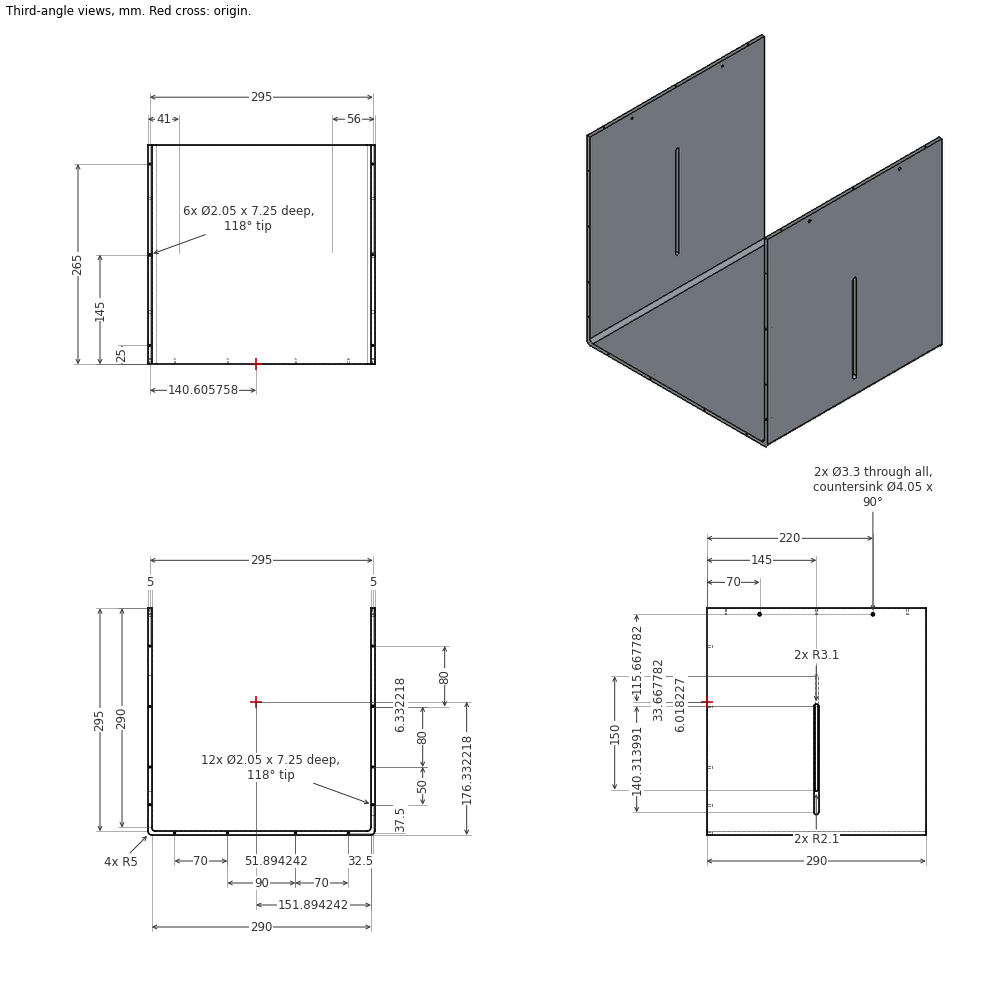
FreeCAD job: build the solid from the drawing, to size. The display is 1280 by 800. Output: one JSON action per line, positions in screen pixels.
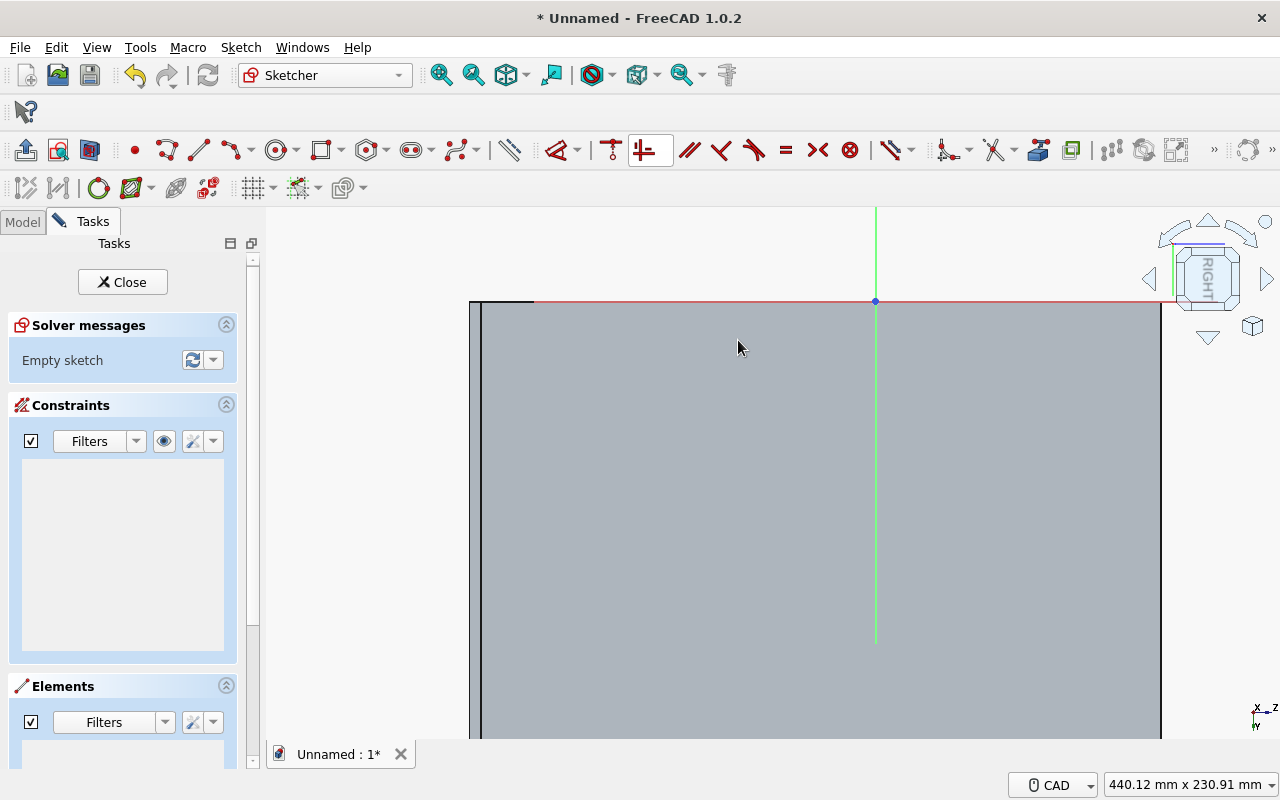
{"action": "left_click", "coordinate": [412, 150]}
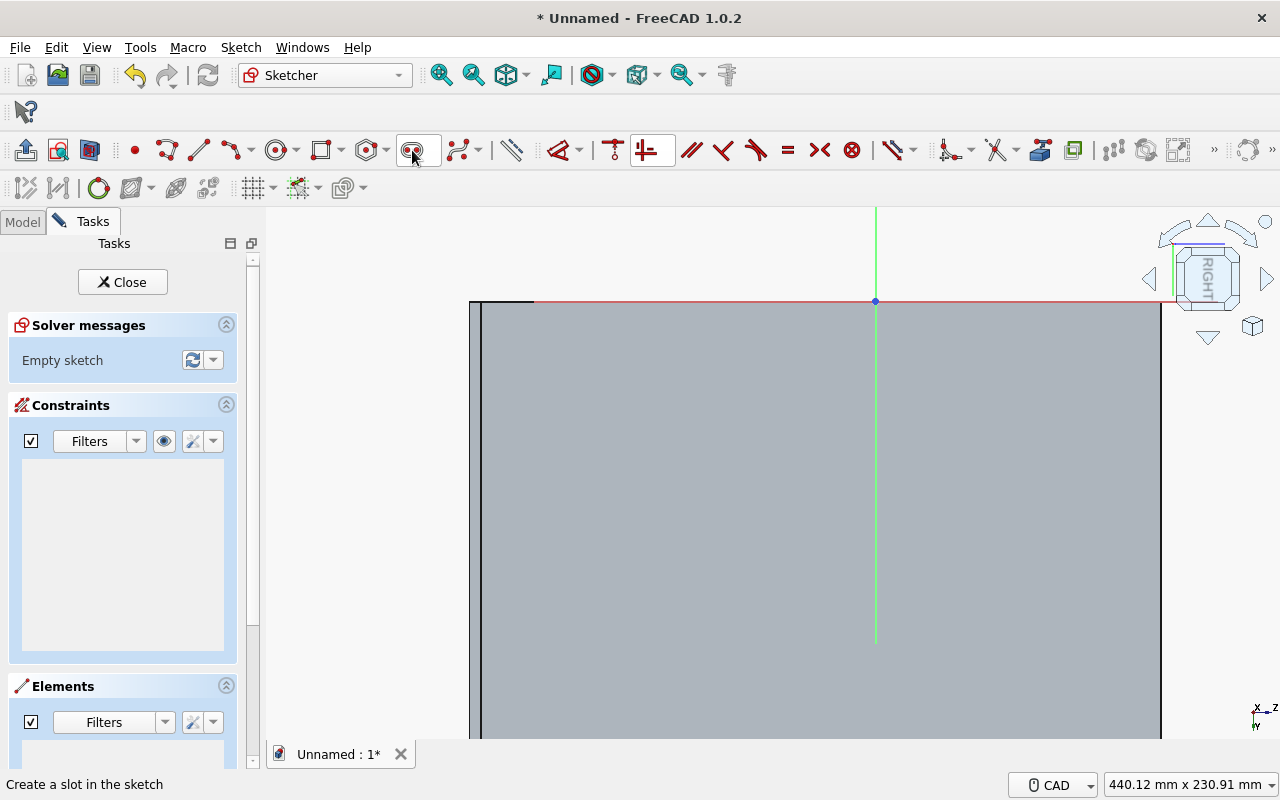
{"action": "scroll", "coordinate": [539, 636], "scroll_direction": "up", "scroll_amount": 6}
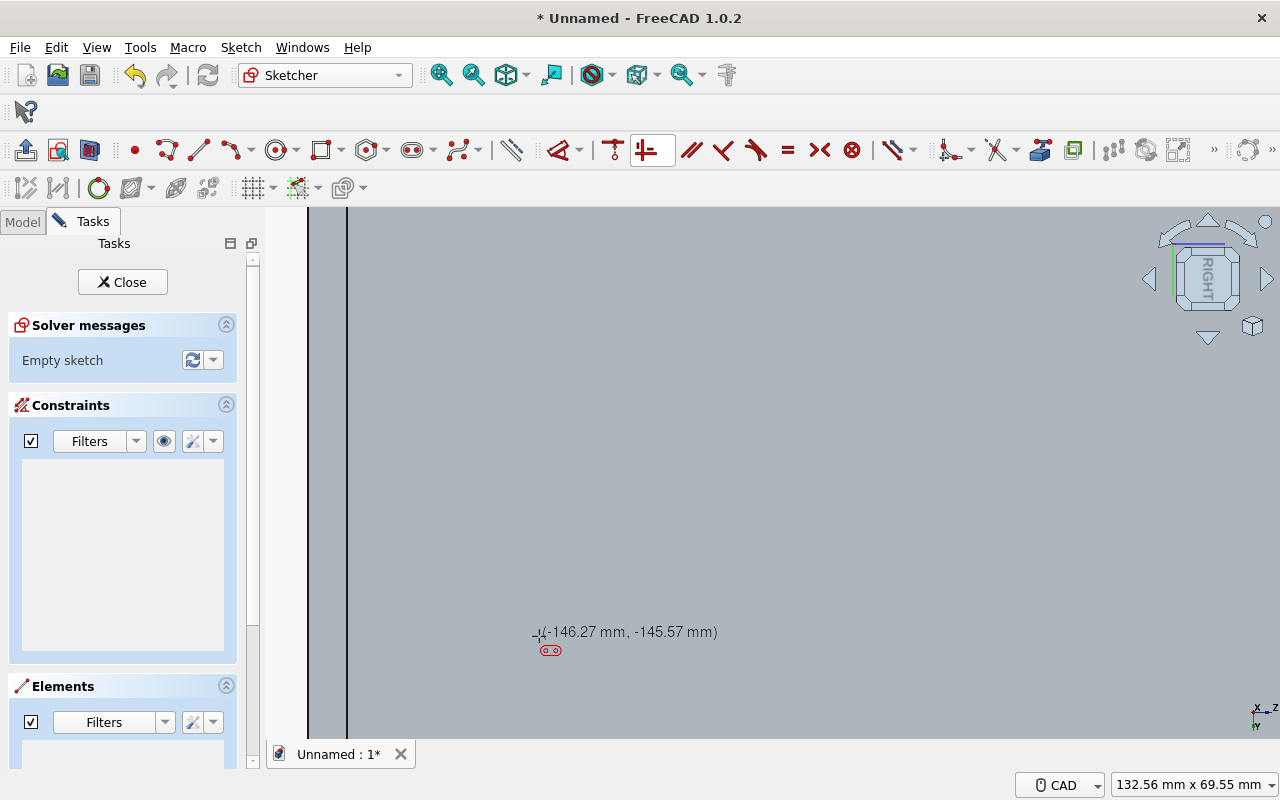
{"action": "left_click", "coordinate": [538, 633]}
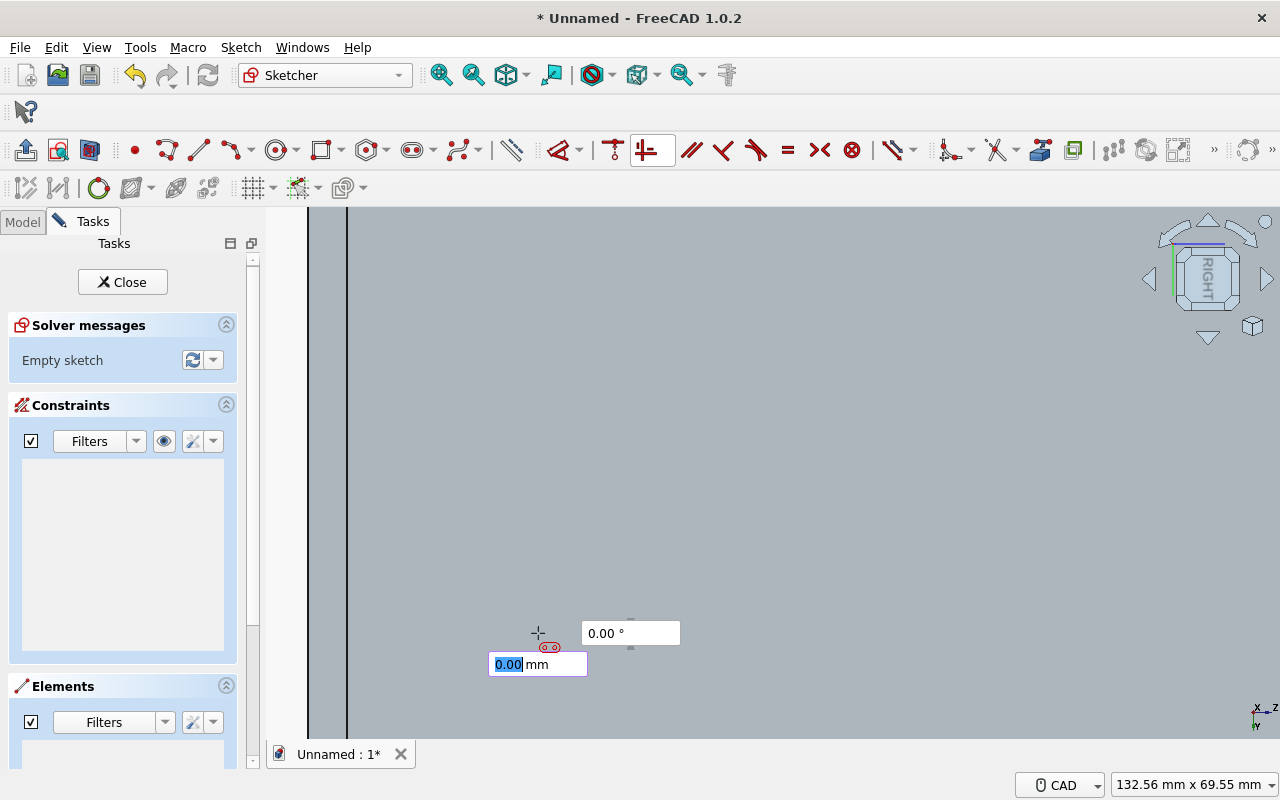
{"action": "scroll", "coordinate": [540, 638], "scroll_direction": "down", "scroll_amount": 6}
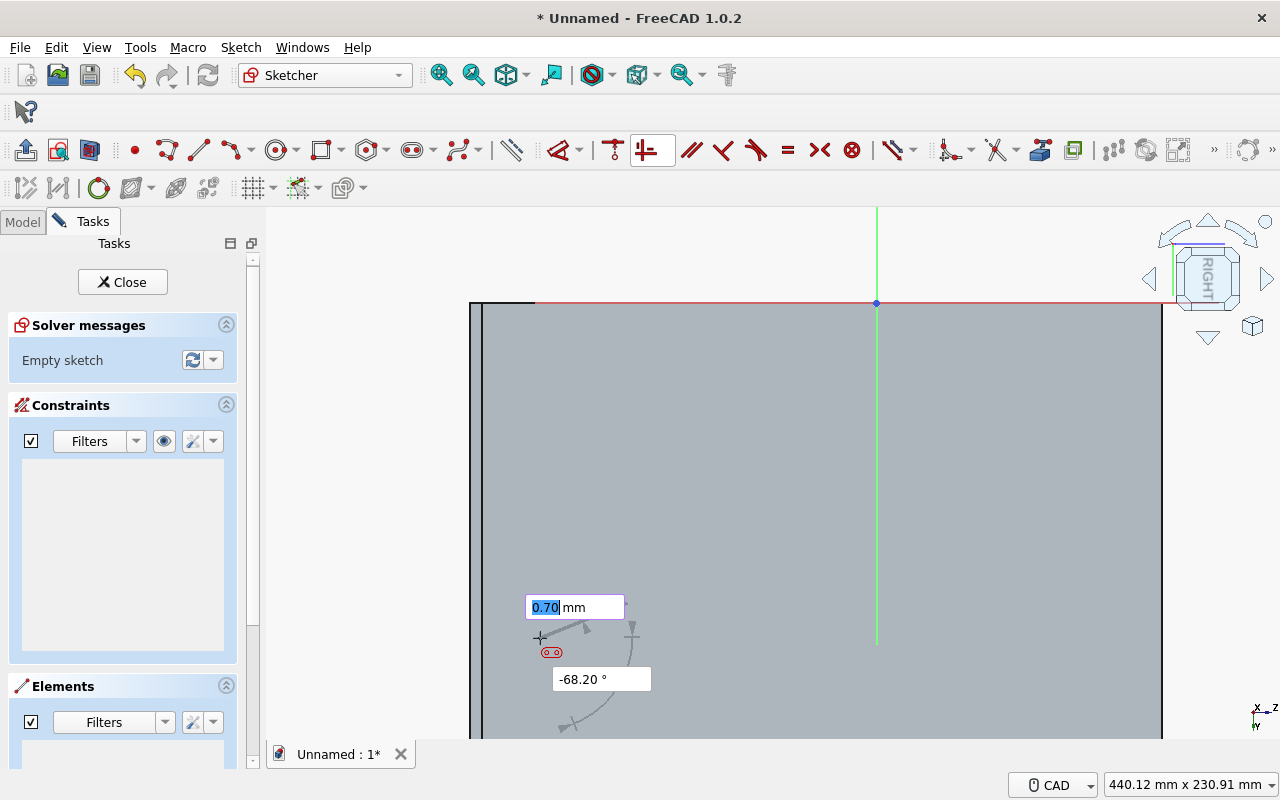
{"action": "left_click", "coordinate": [863, 637]}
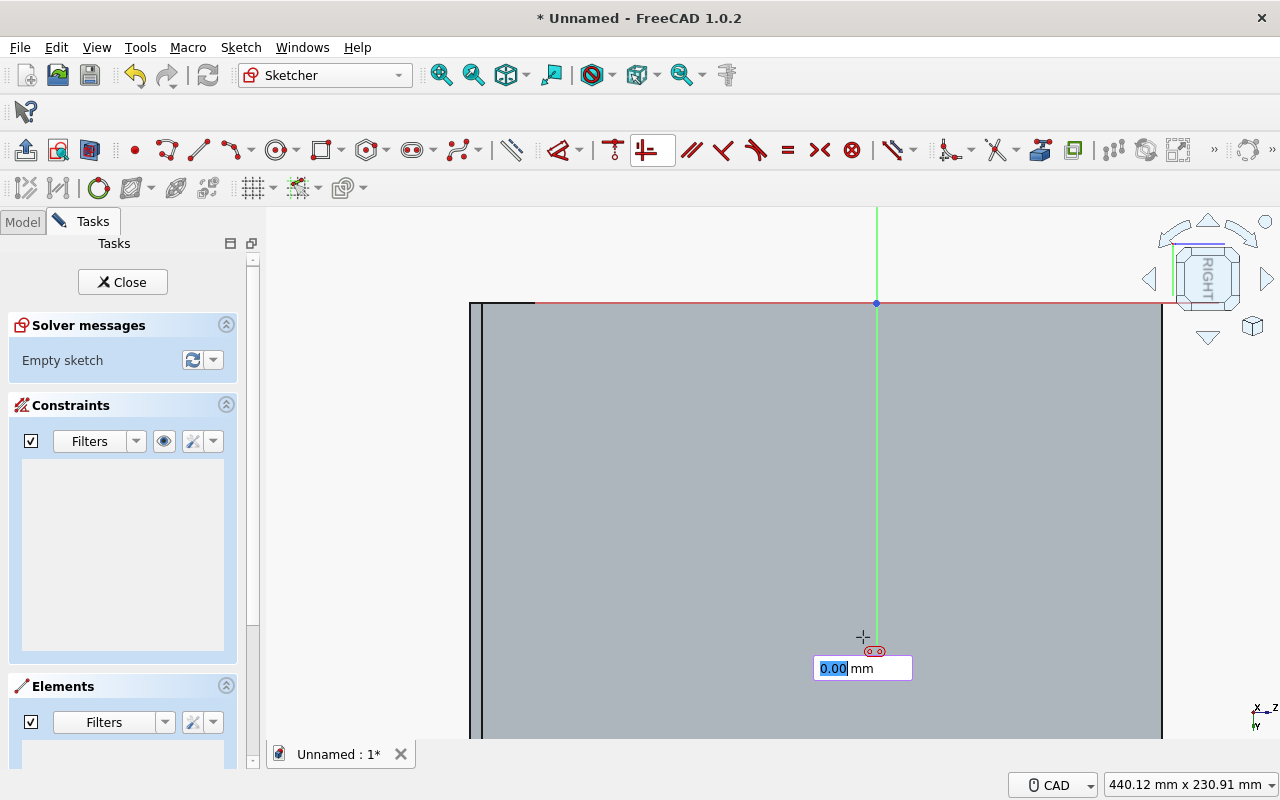
{"action": "scroll", "coordinate": [701, 644], "scroll_direction": "up", "scroll_amount": 4}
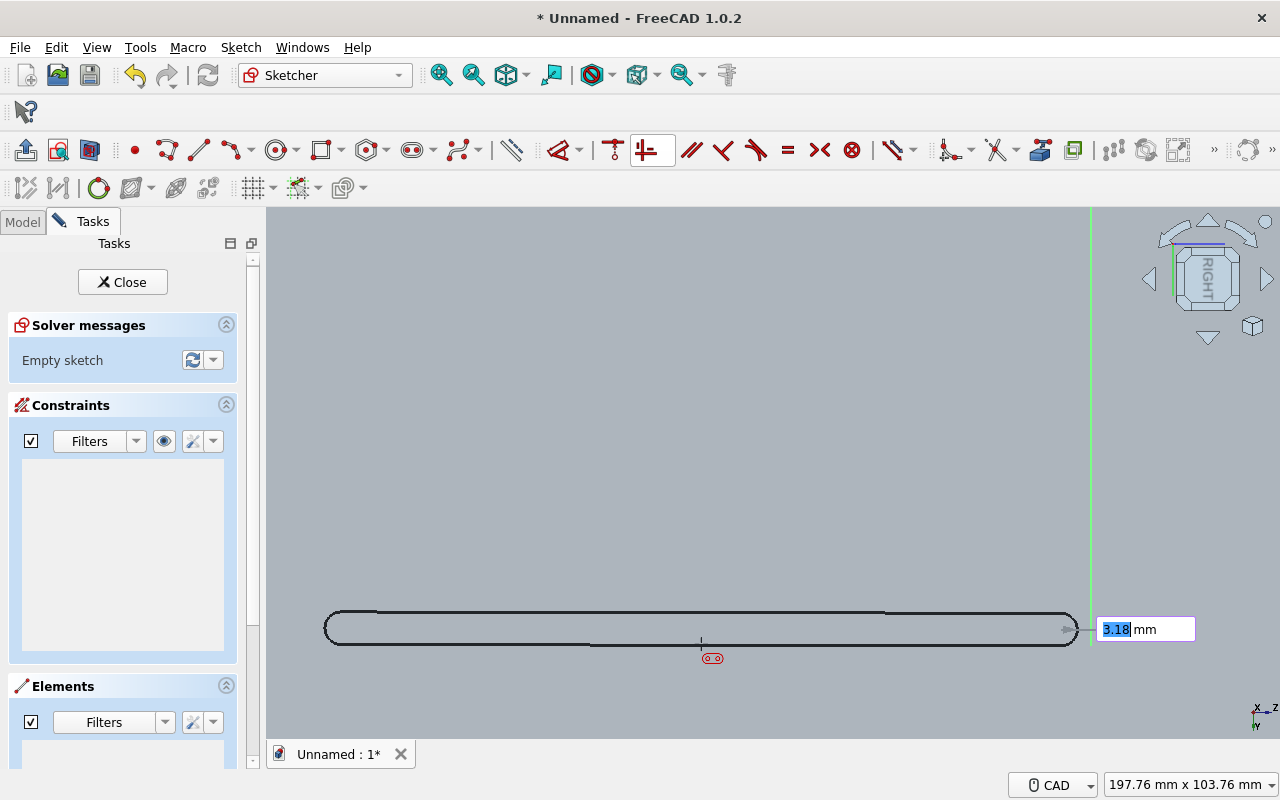
{"action": "left_click", "coordinate": [701, 644]}
{"action": "key", "text": "Escape"}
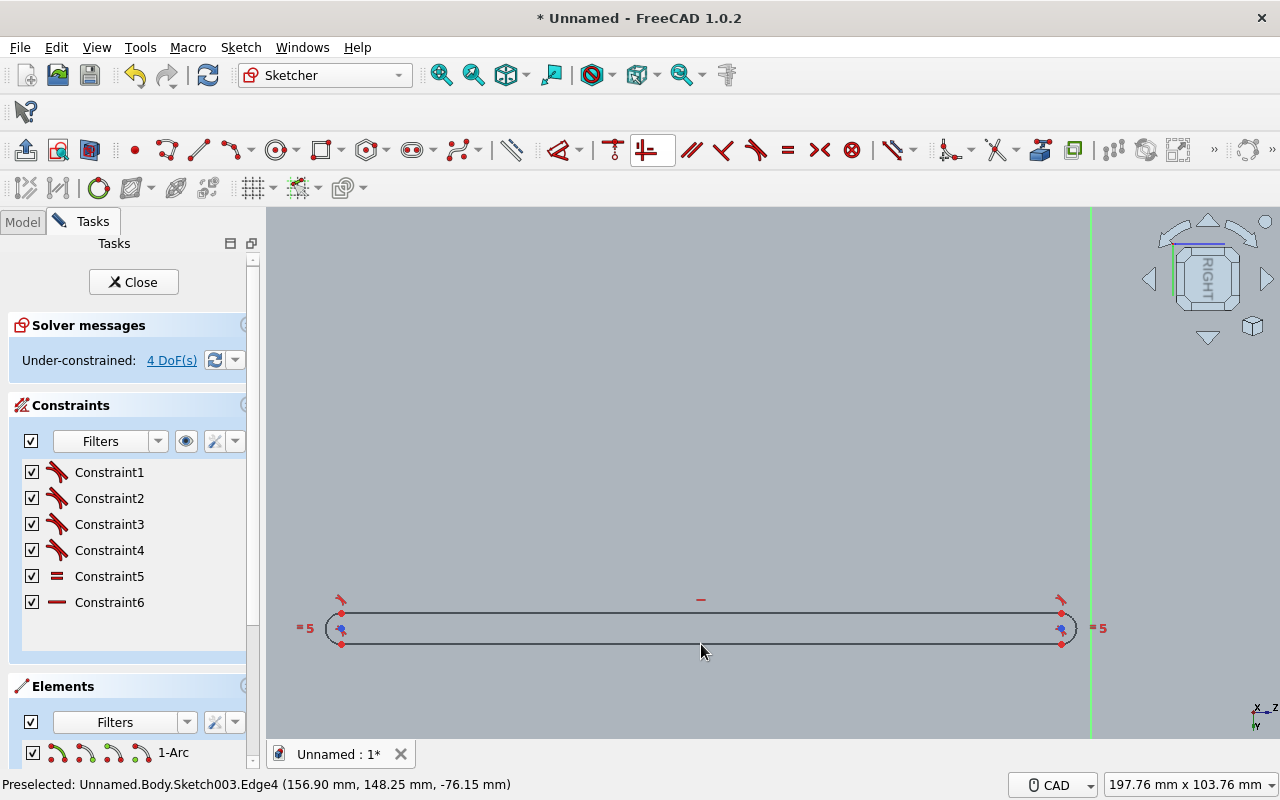
{"action": "left_click", "coordinate": [558, 150]}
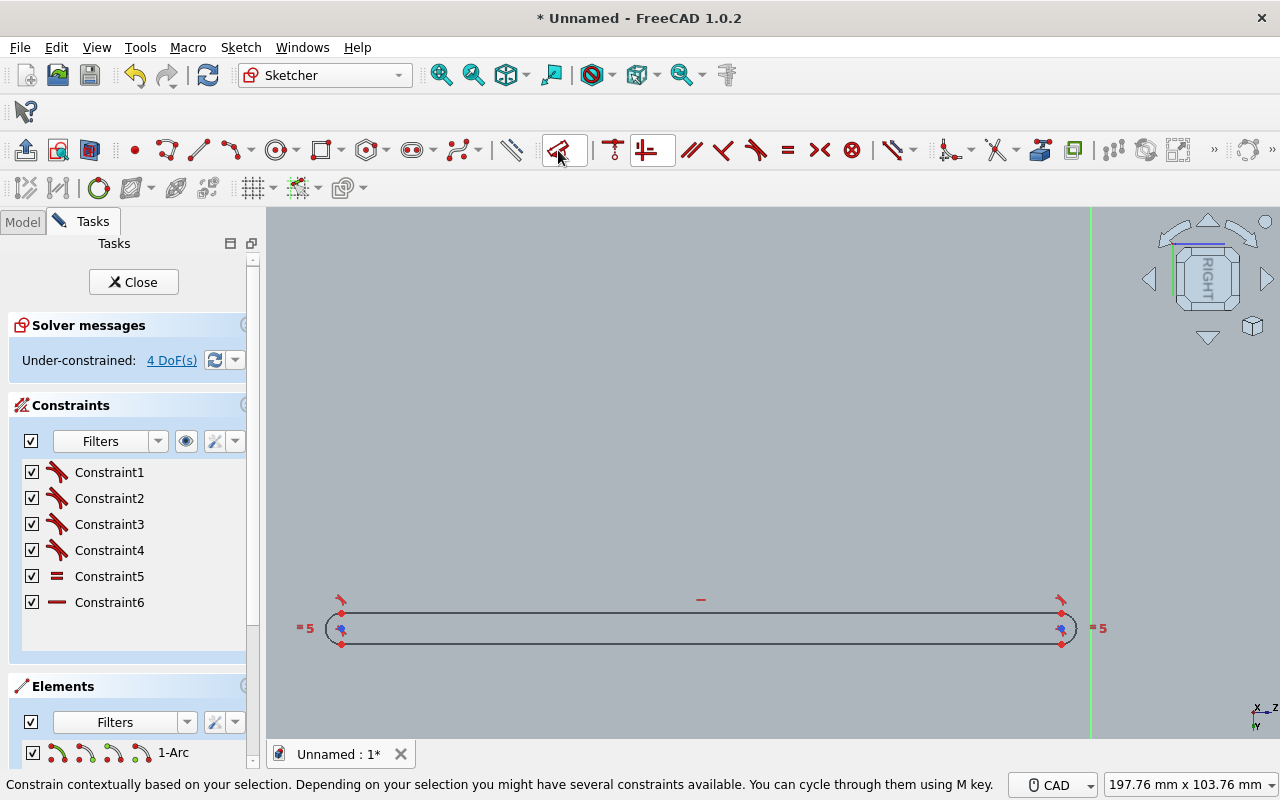
{"action": "scroll", "coordinate": [329, 620], "scroll_direction": "up", "scroll_amount": 5}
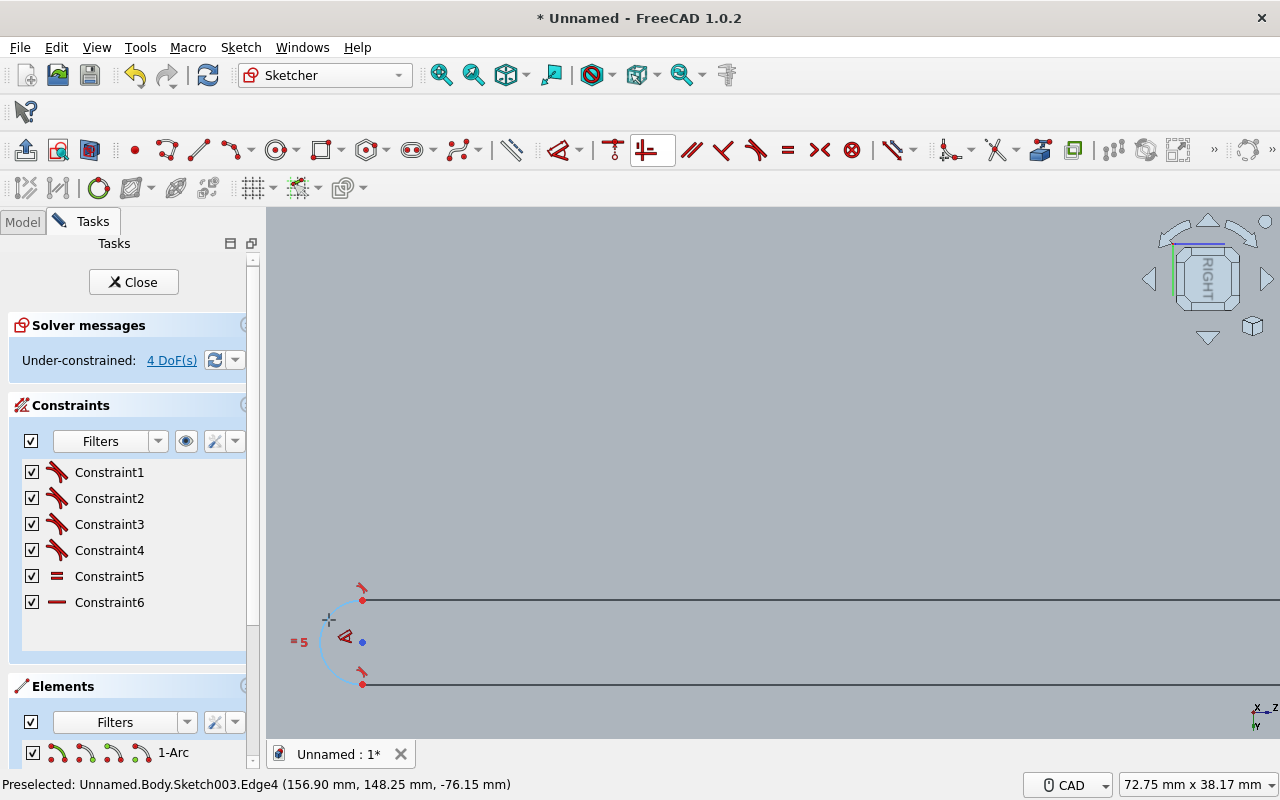
{"action": "left_click", "coordinate": [328, 618]}
{"action": "left_click", "coordinate": [302, 599]}